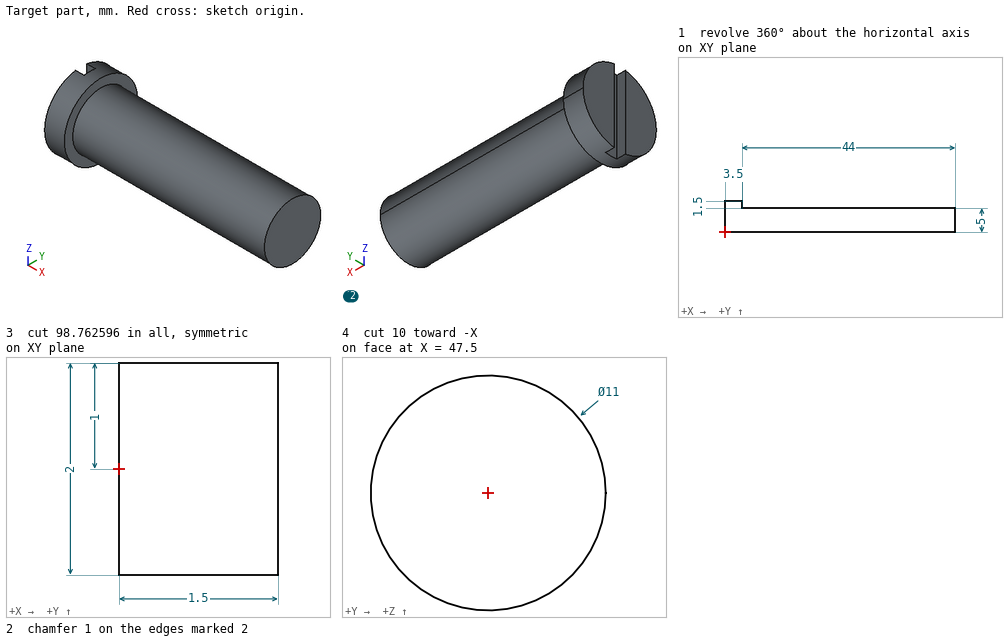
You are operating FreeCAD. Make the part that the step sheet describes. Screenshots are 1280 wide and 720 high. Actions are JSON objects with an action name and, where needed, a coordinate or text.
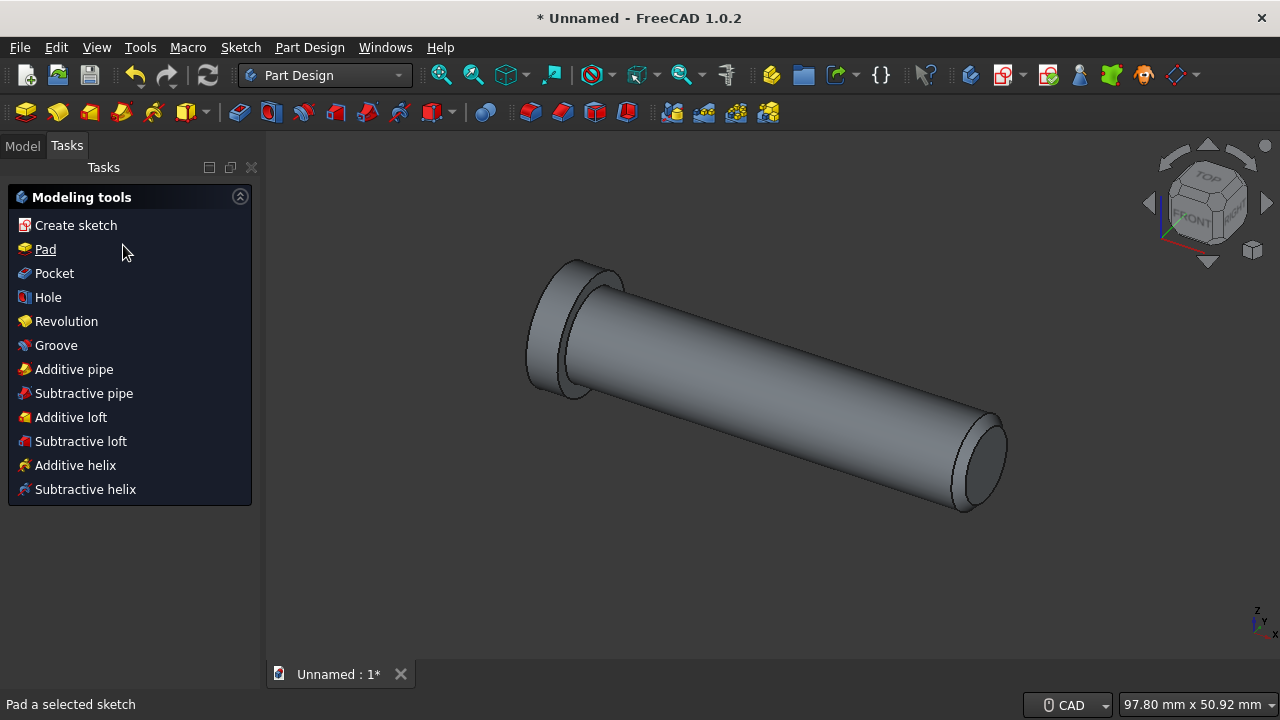
{"action": "left_click", "coordinate": [240, 112]}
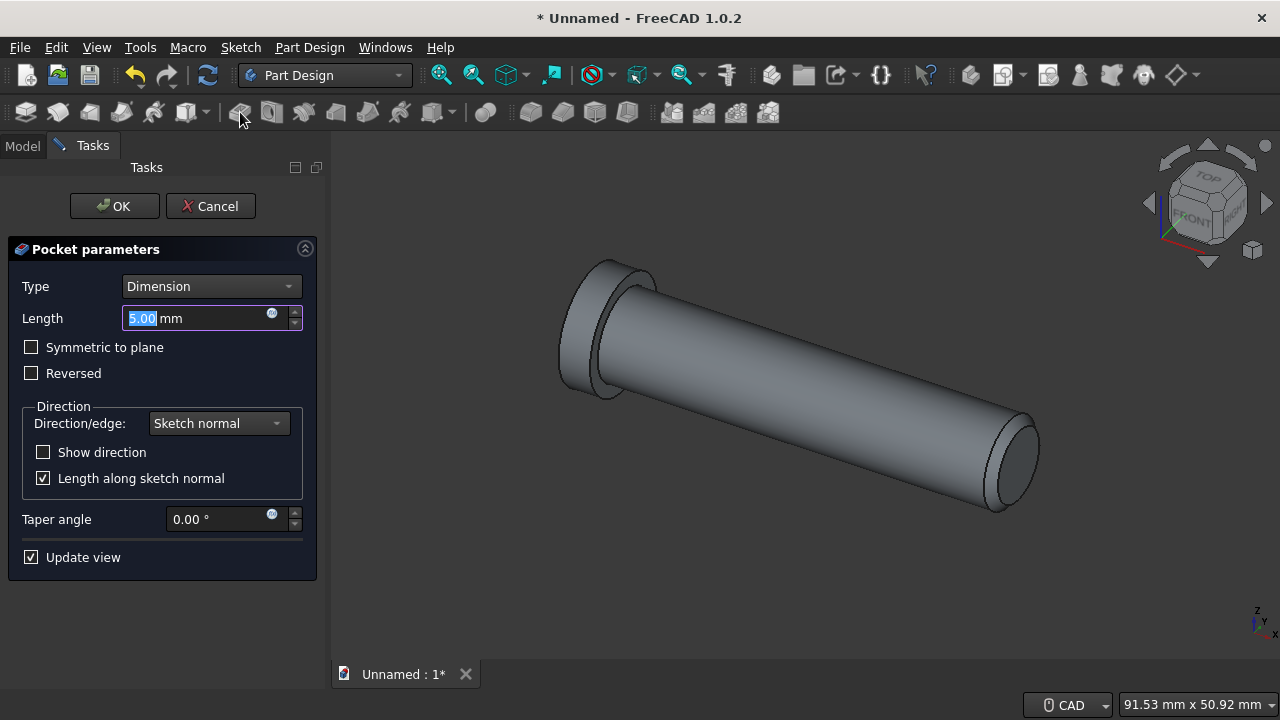
{"action": "type", "text": "98.762596"}
{"action": "key", "text": "Tab"}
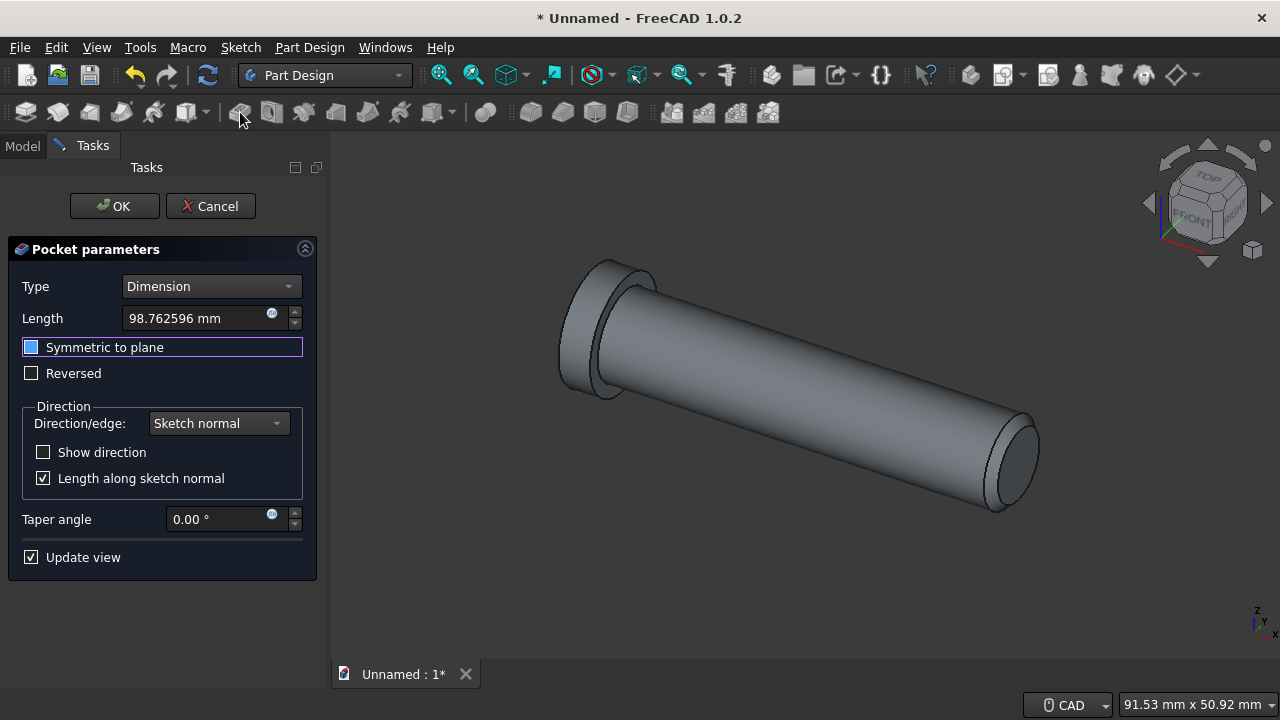
{"action": "left_click", "coordinate": [30, 347]}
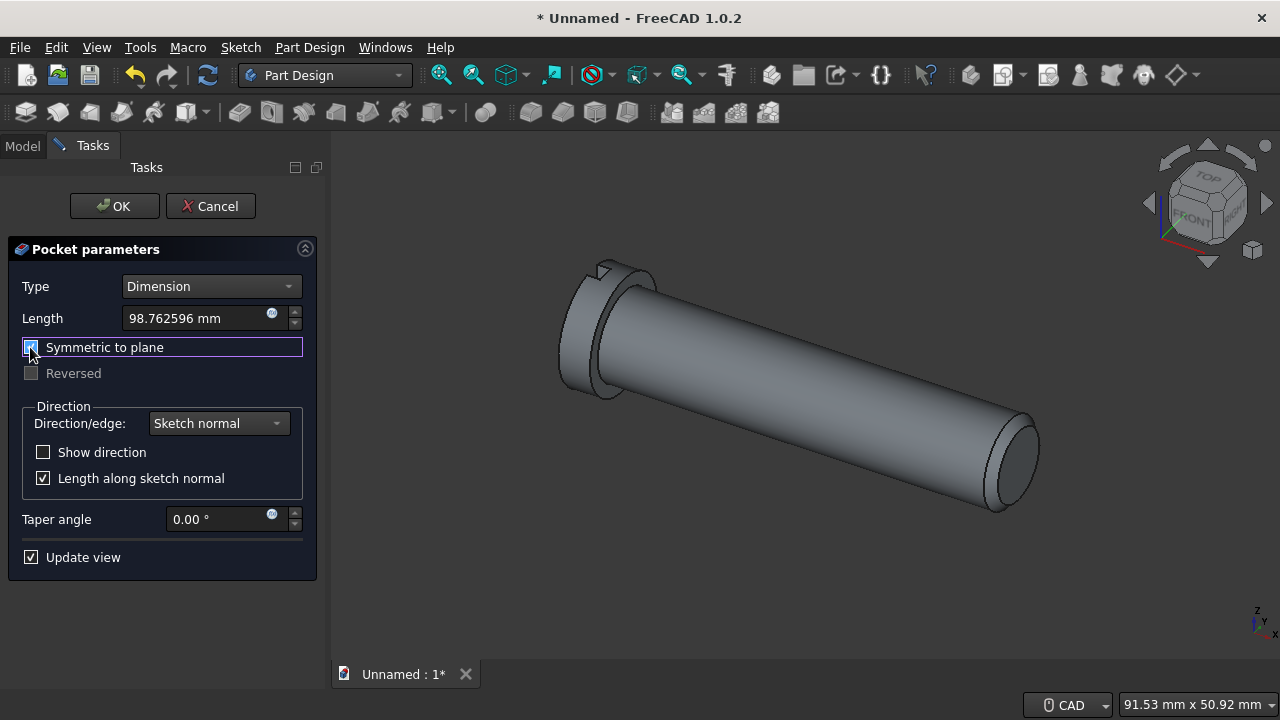
{"action": "left_click", "coordinate": [115, 206]}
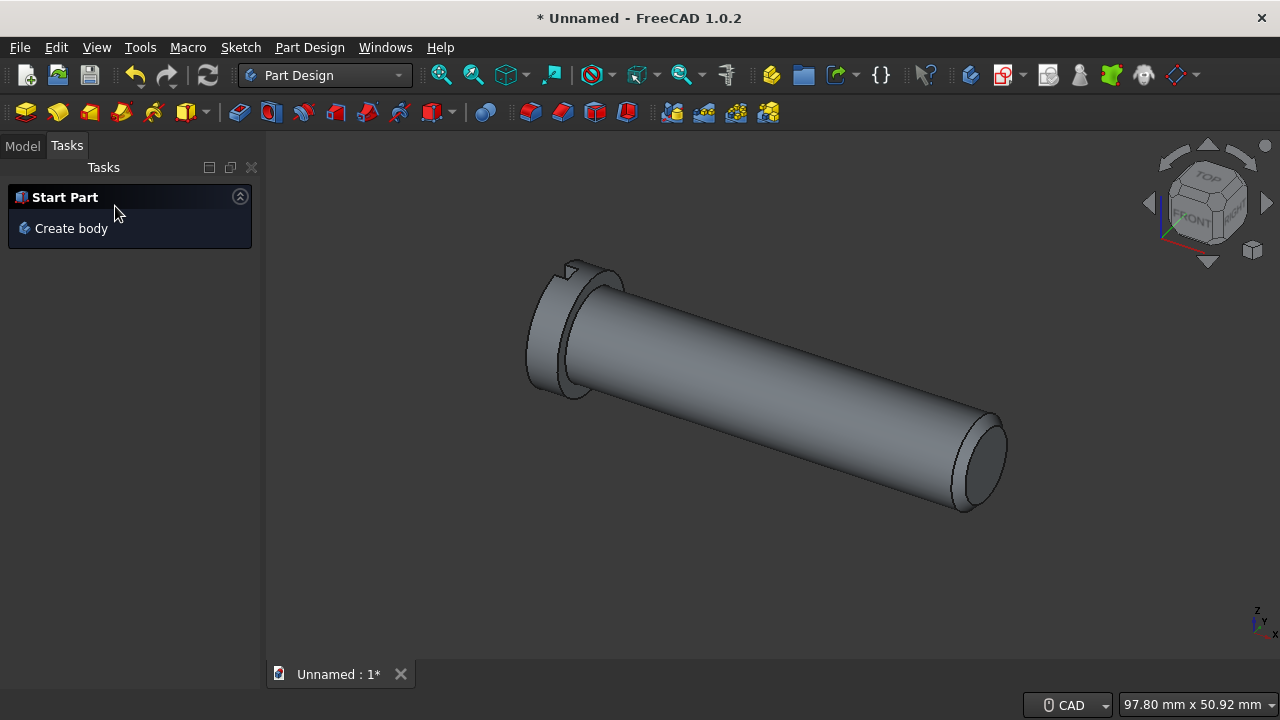
{"action": "left_click", "coordinate": [986, 465]}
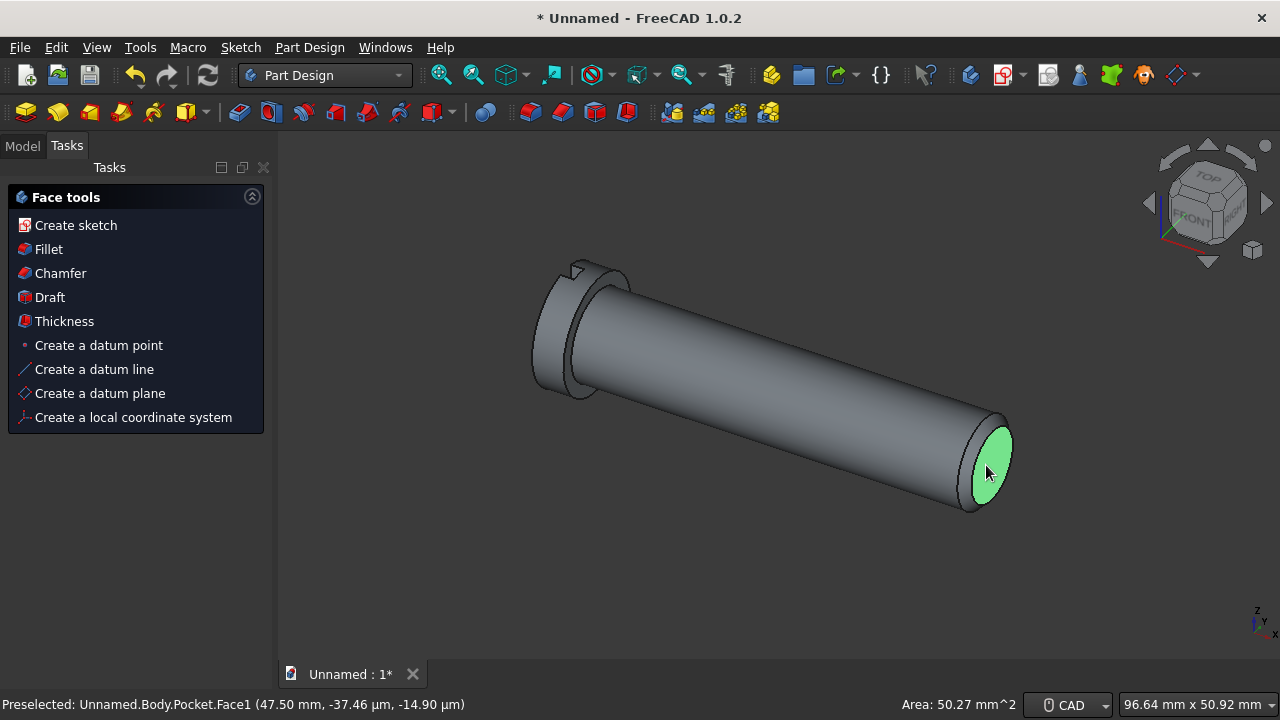
{"action": "left_click", "coordinate": [1004, 76]}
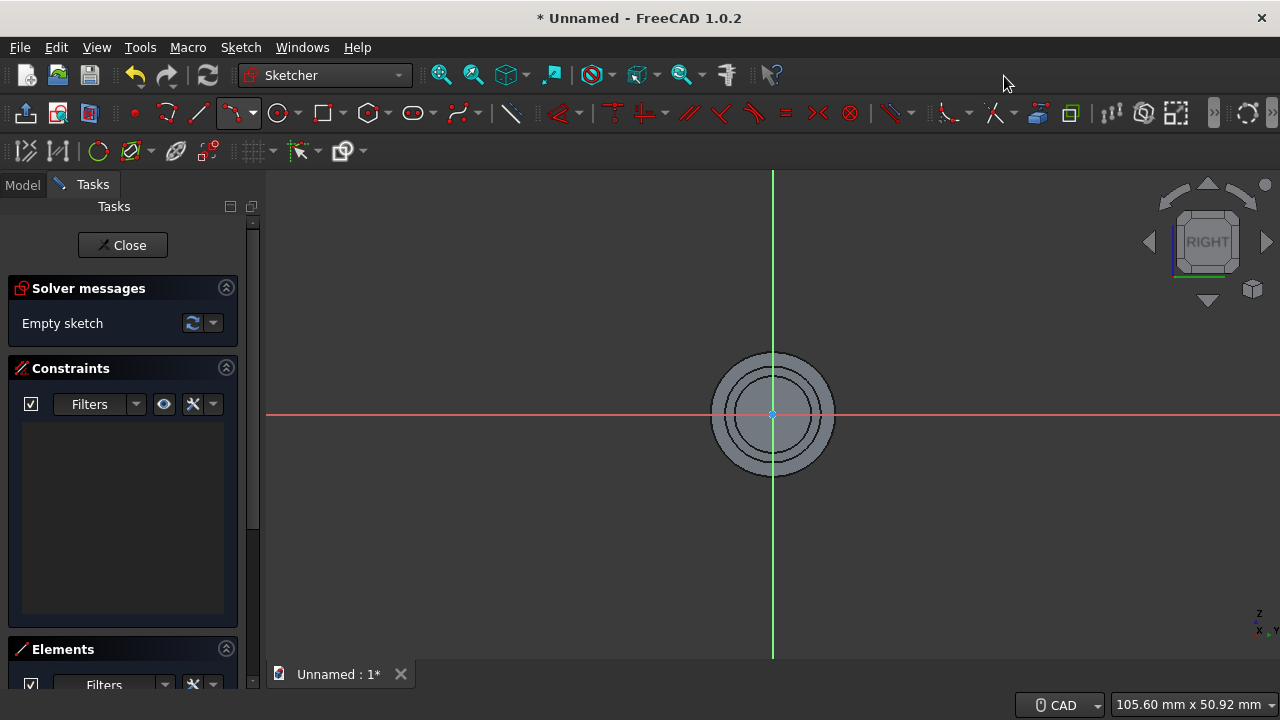
{"action": "scroll", "coordinate": [813, 415], "scroll_direction": "up", "scroll_amount": 5}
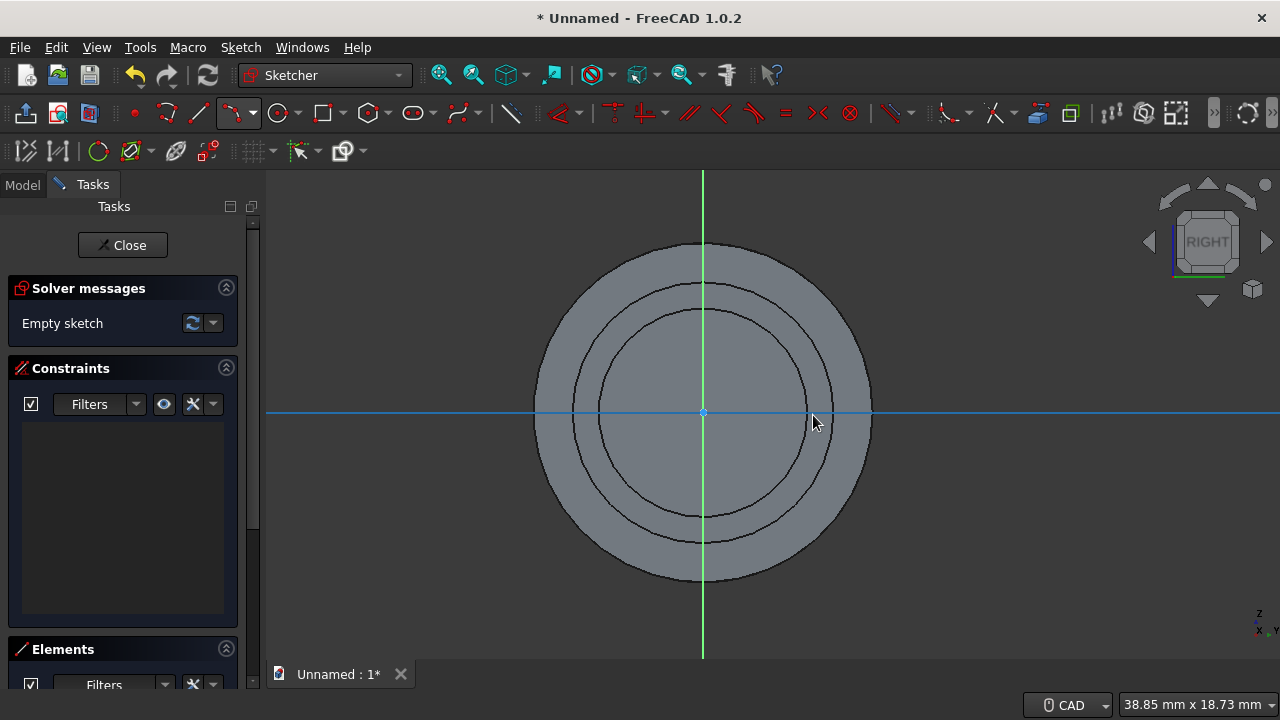
{"action": "key", "text": "g c"}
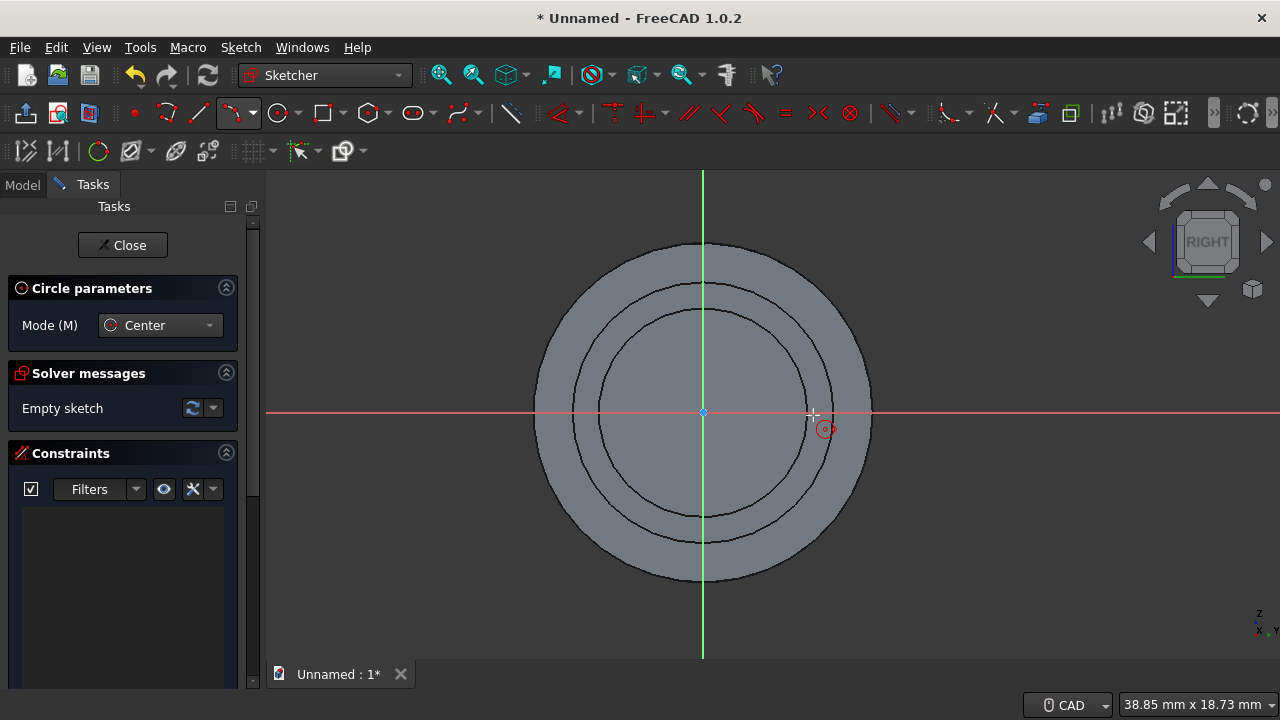
{"action": "left_click", "coordinate": [703, 413]}
{"action": "left_click", "coordinate": [805, 311]}
{"action": "key", "text": "Escape"}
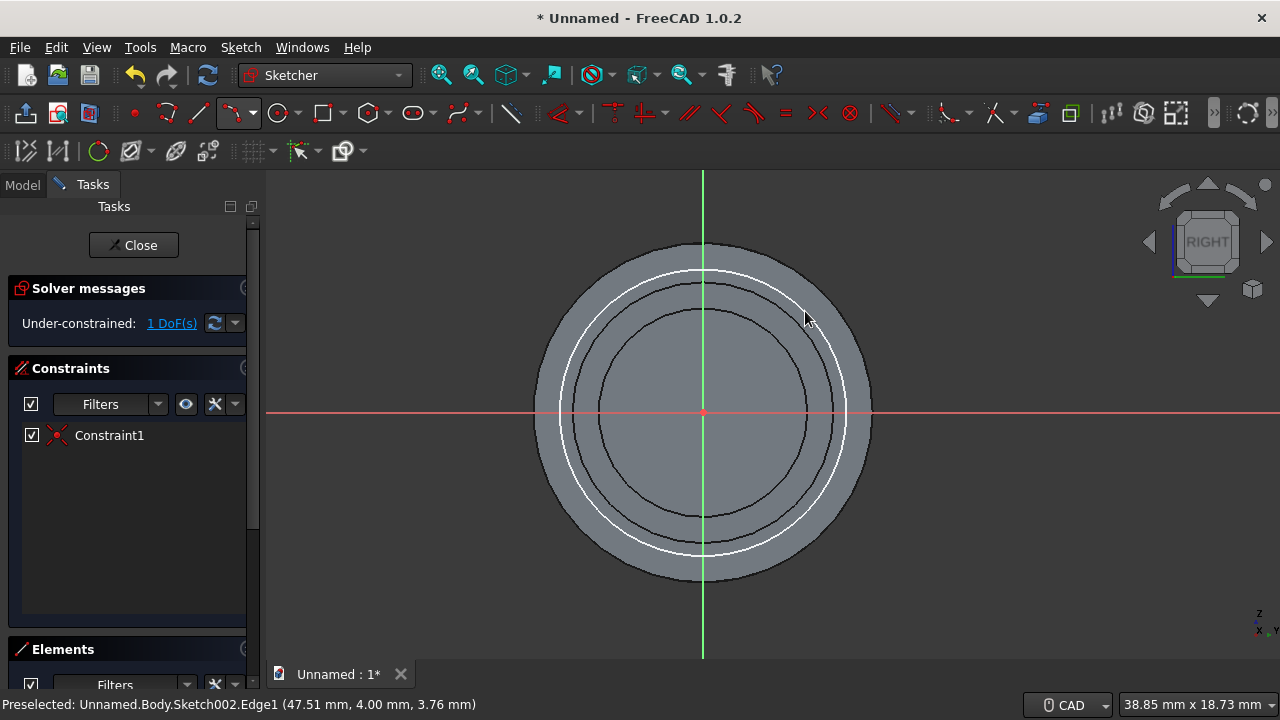
{"action": "key", "text": "d"}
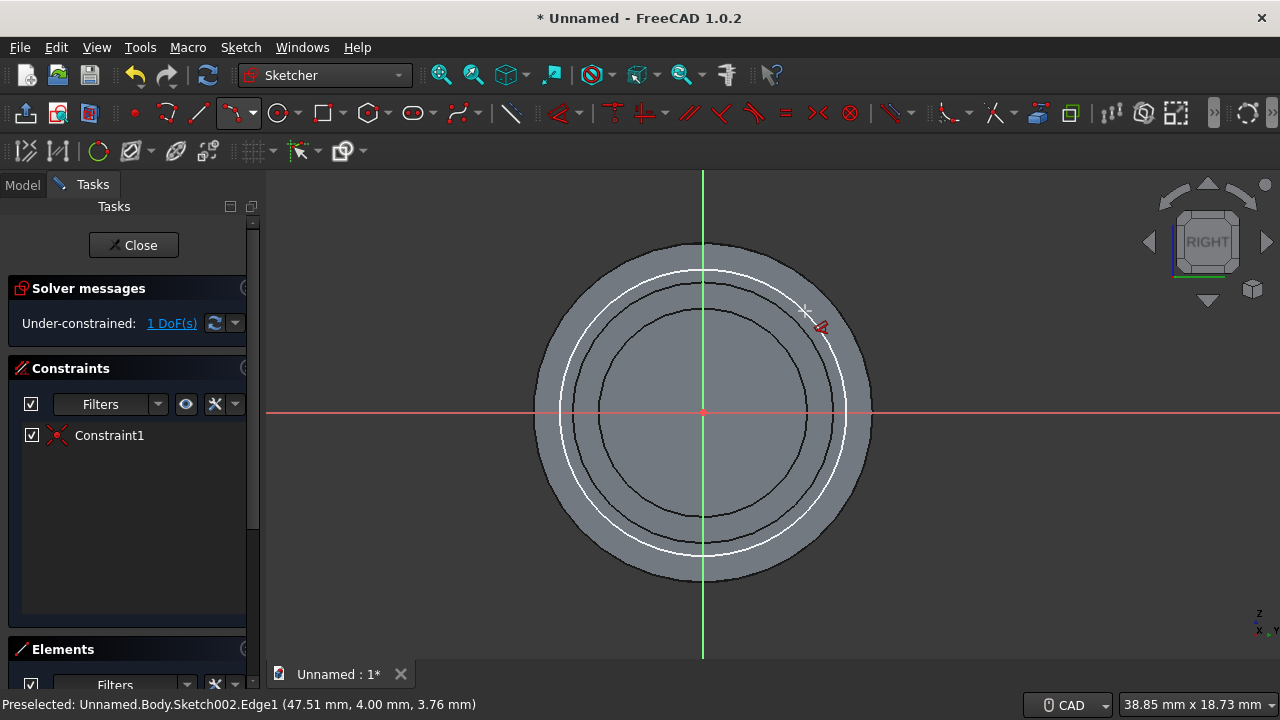
{"action": "left_click", "coordinate": [804, 311]}
{"action": "left_click", "coordinate": [827, 288]}